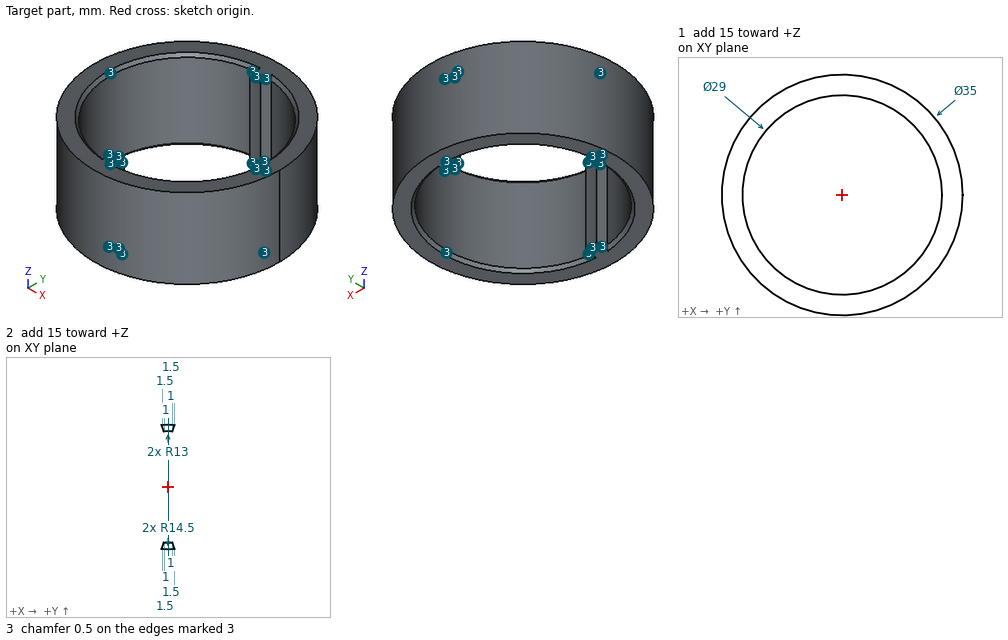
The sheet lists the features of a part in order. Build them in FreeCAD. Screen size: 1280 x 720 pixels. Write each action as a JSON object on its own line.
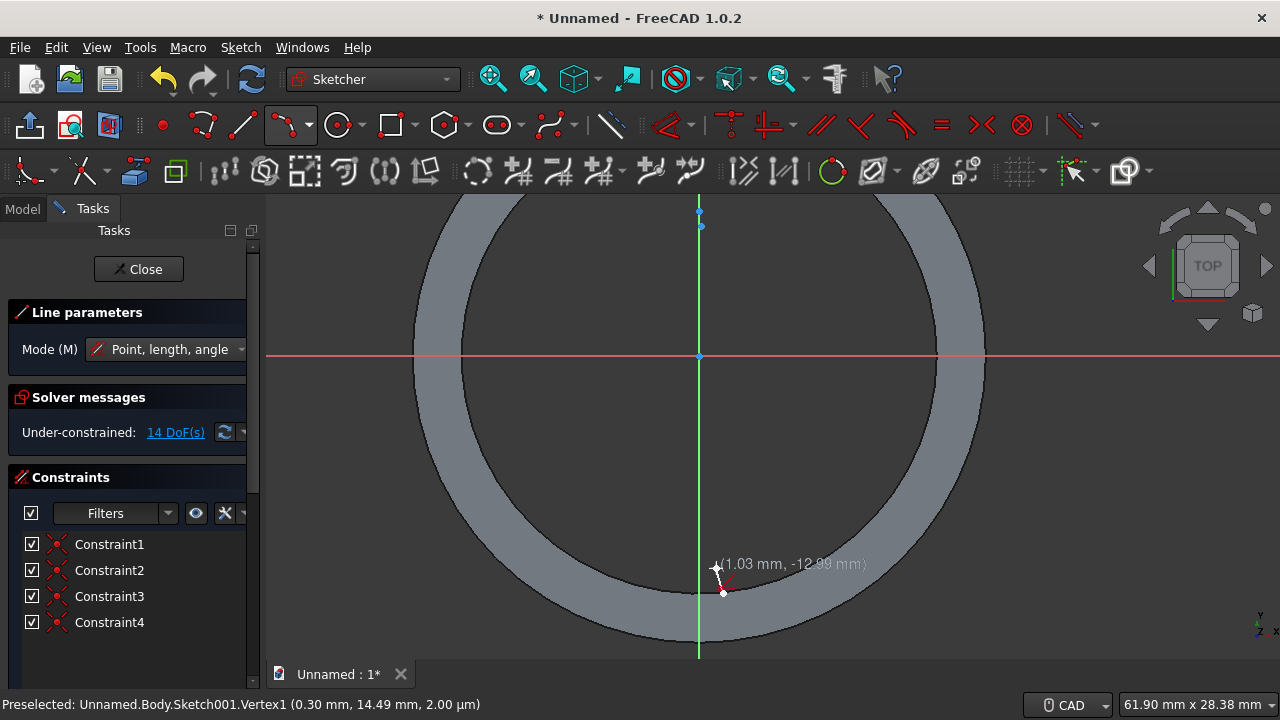
{"action": "left_click", "coordinate": [683, 568]}
{"action": "left_click", "coordinate": [675, 592]}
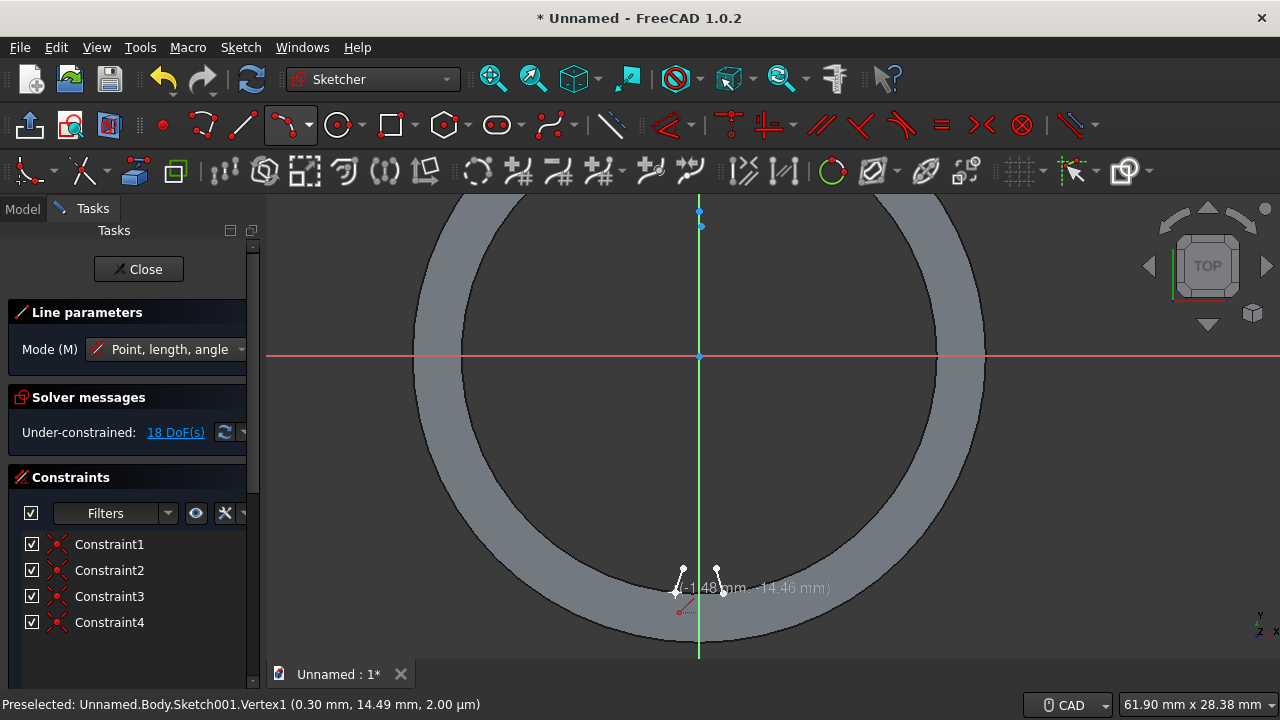
{"action": "left_click", "coordinate": [284, 126]}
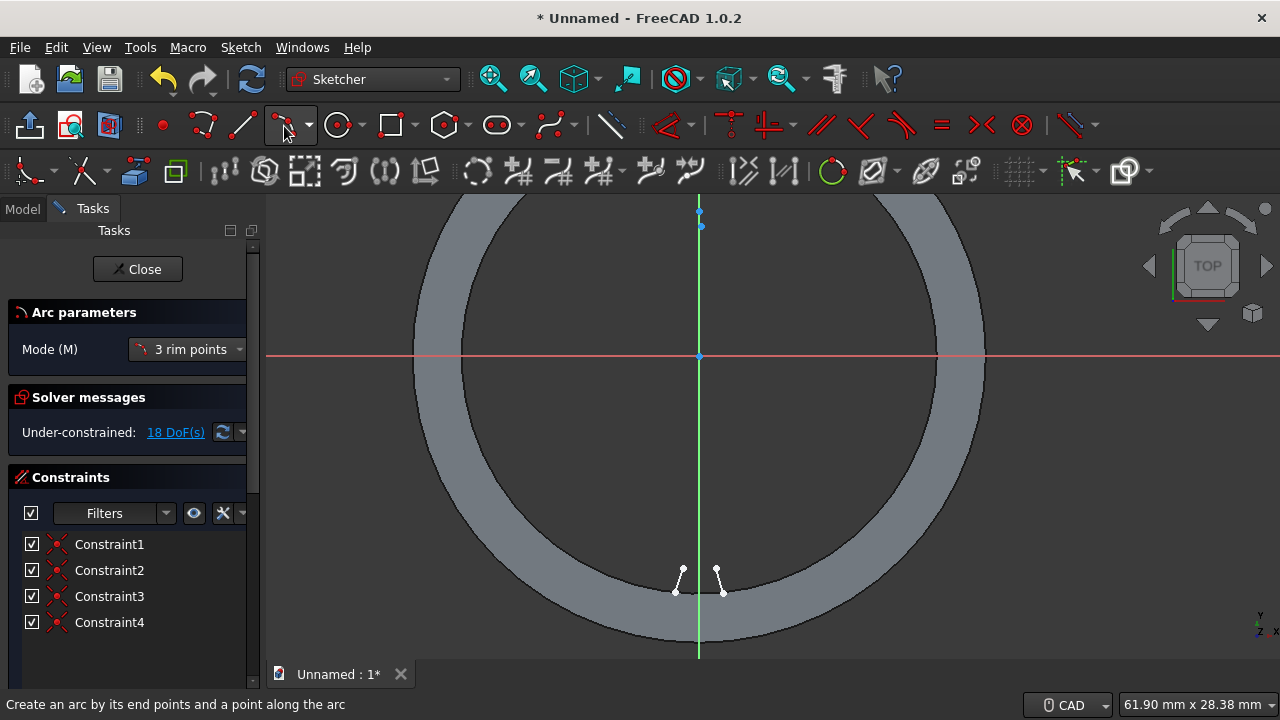
{"action": "scroll", "coordinate": [716, 568], "scroll_direction": "up", "scroll_amount": 2}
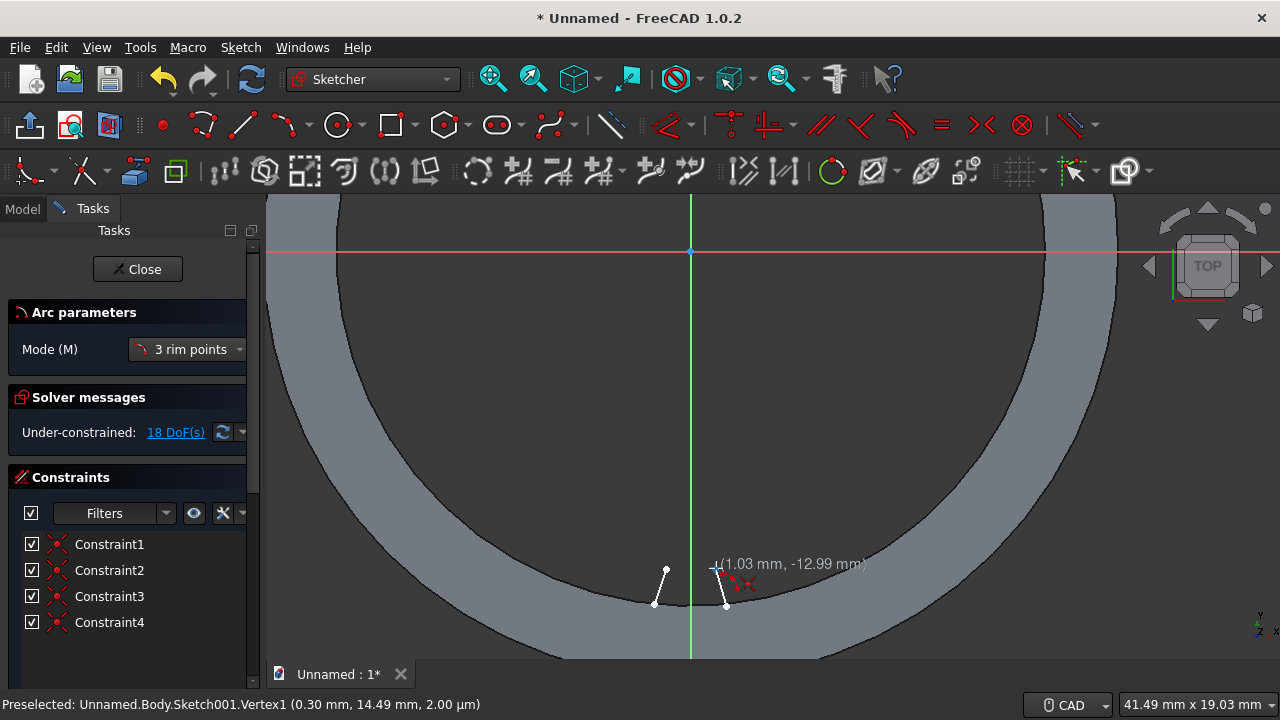
{"action": "left_click", "coordinate": [716, 569]}
{"action": "left_click", "coordinate": [667, 569]}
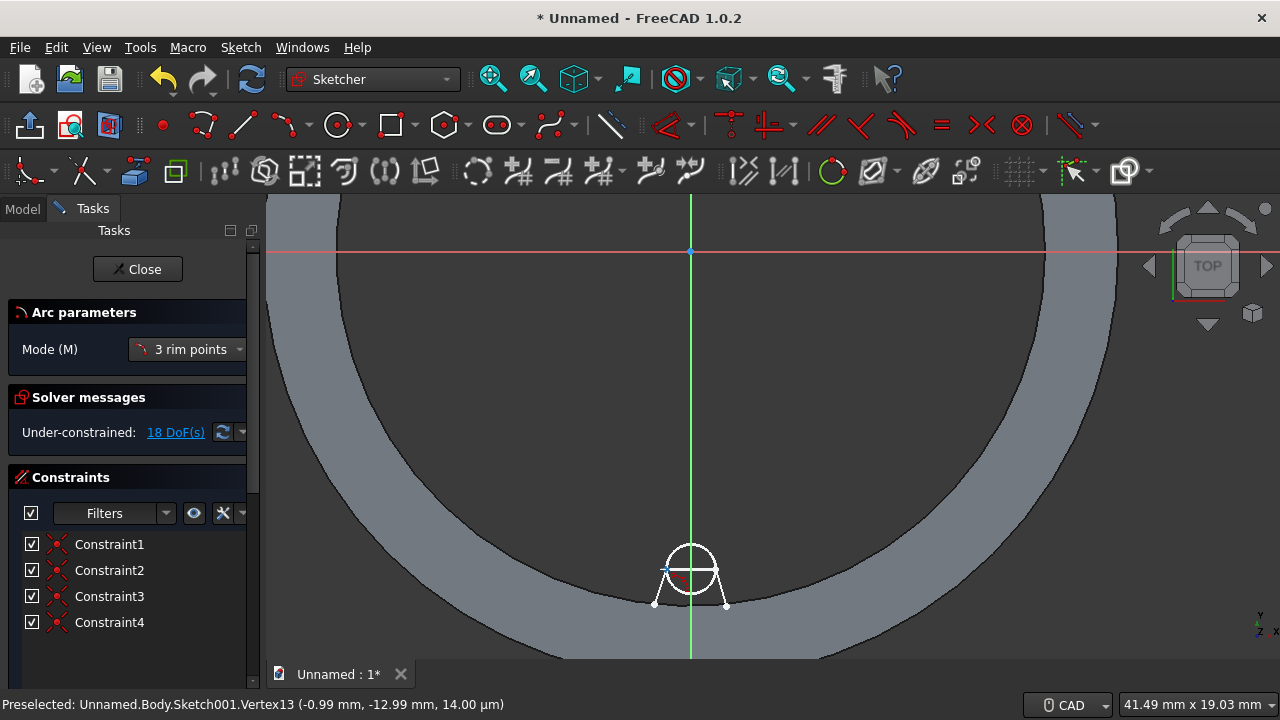
{"action": "scroll", "coordinate": [686, 569], "scroll_direction": "up", "scroll_amount": 15}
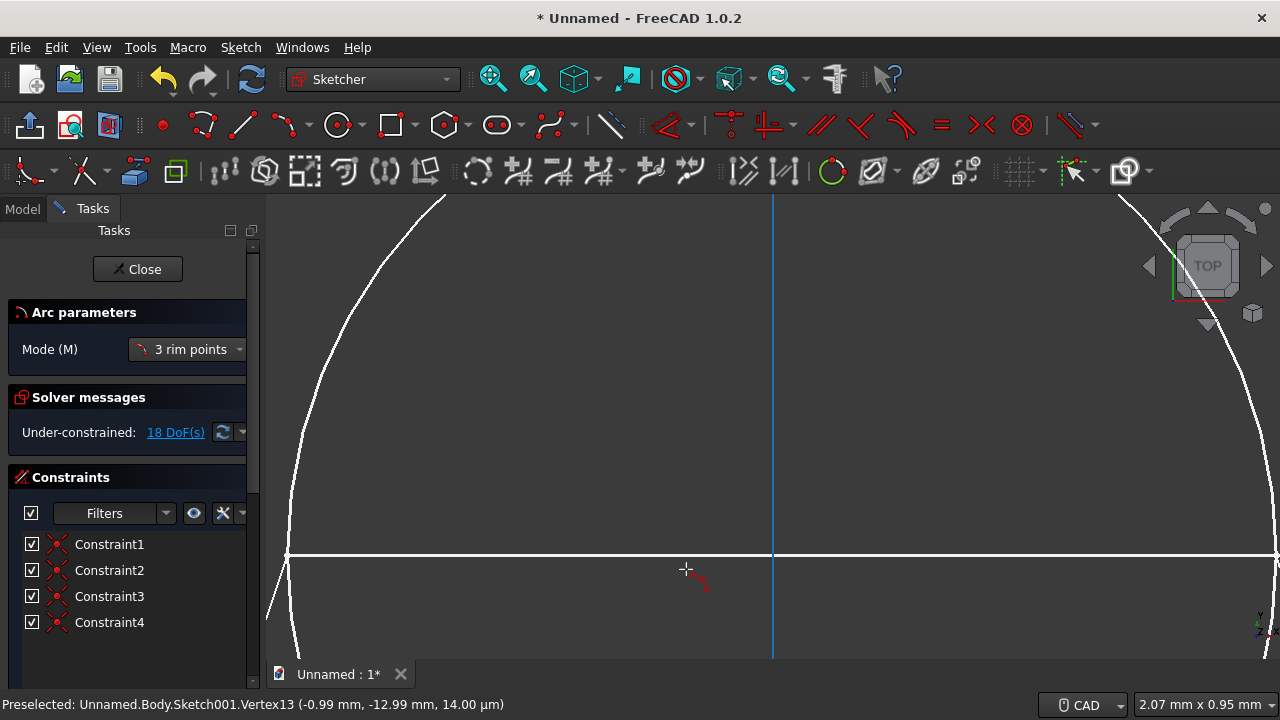
{"action": "left_click", "coordinate": [674, 557]}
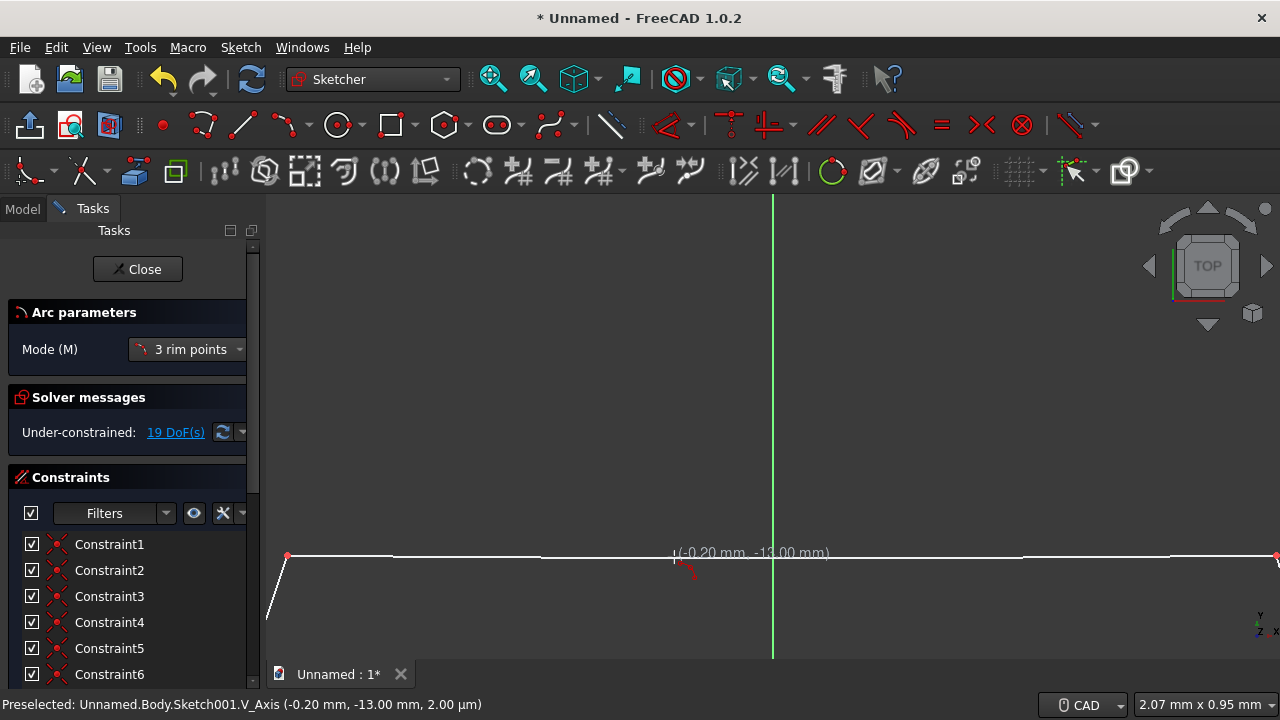
{"action": "scroll", "coordinate": [704, 426], "scroll_direction": "down", "scroll_amount": 15}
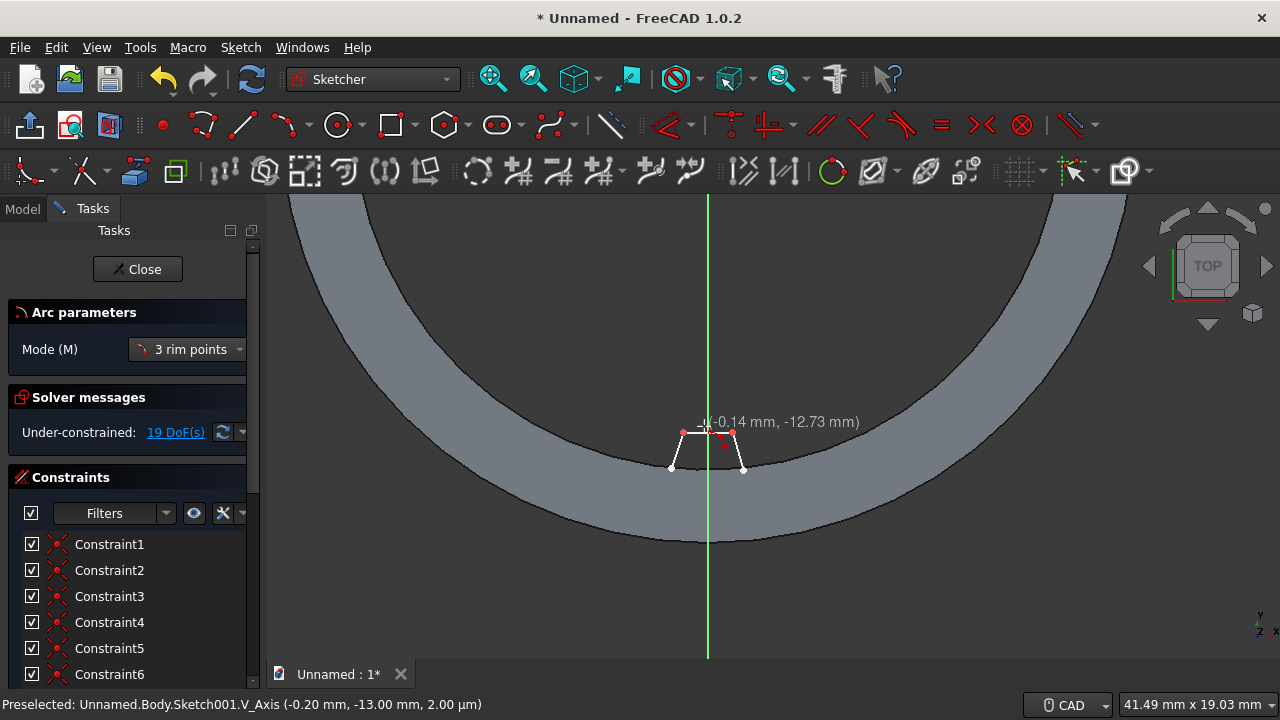
{"action": "scroll", "coordinate": [703, 608], "scroll_direction": "down", "scroll_amount": 5}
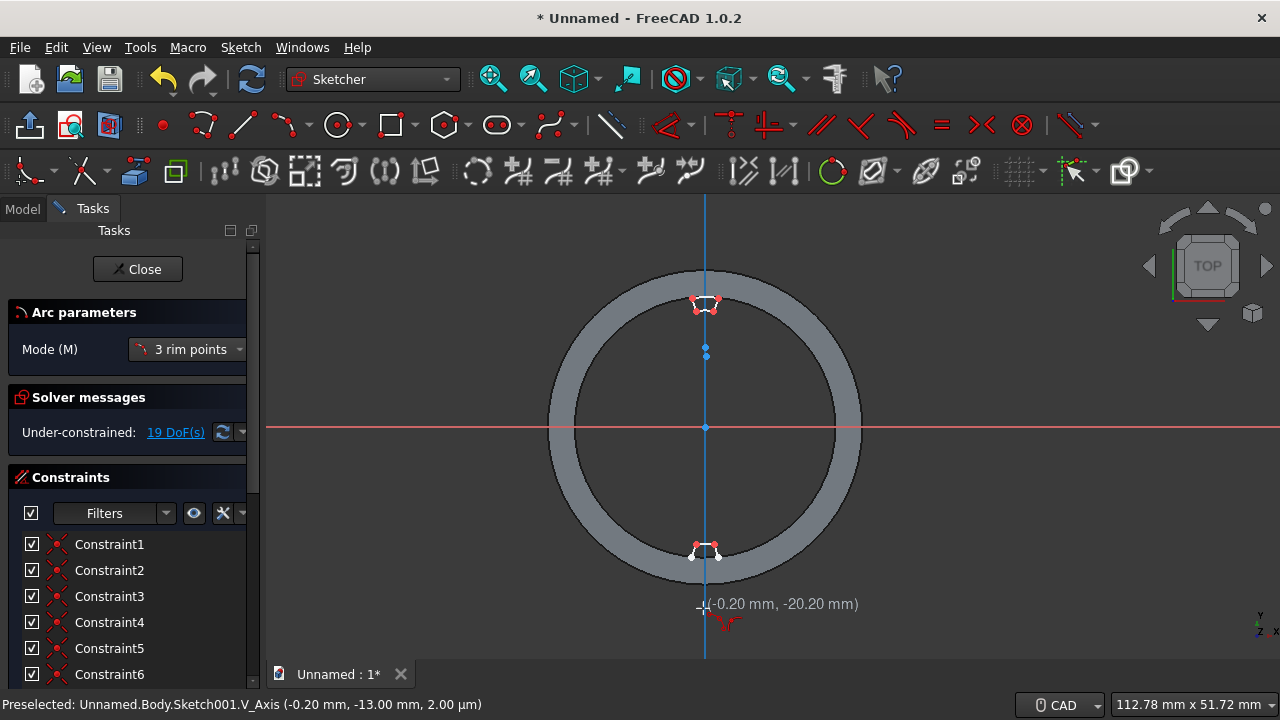
{"action": "scroll", "coordinate": [692, 557], "scroll_direction": "up", "scroll_amount": 5}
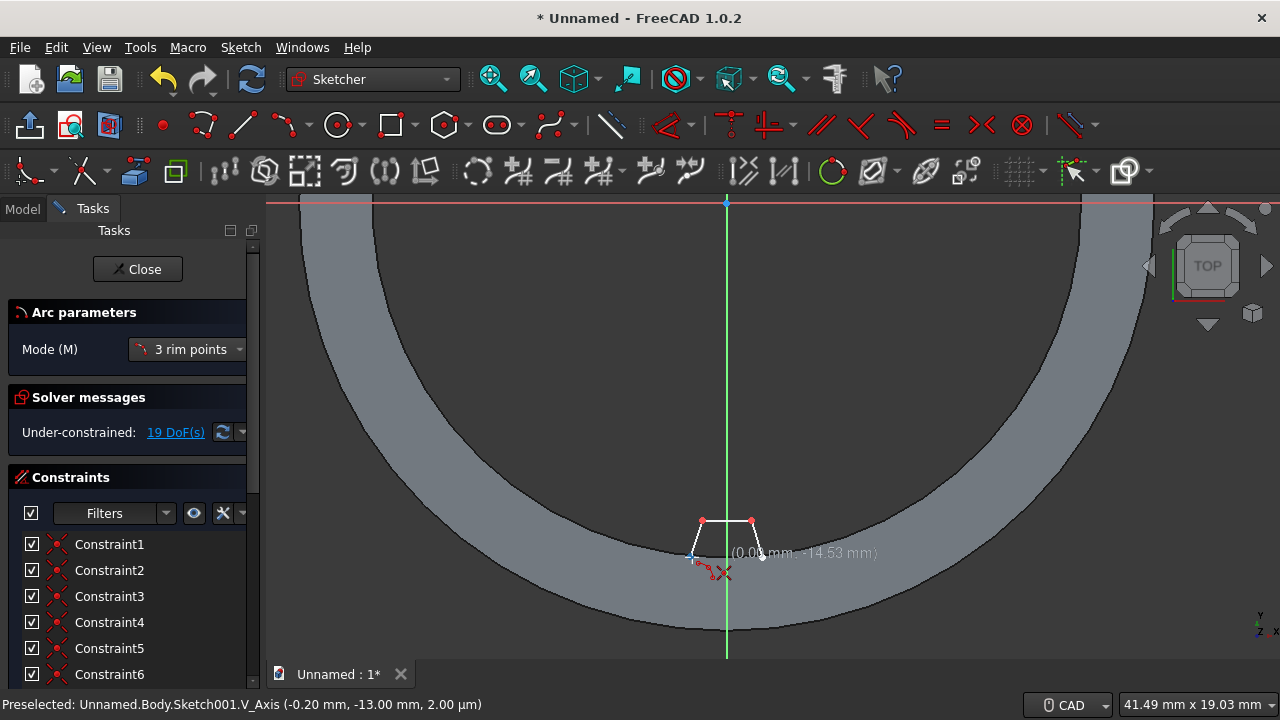
{"action": "left_click", "coordinate": [691, 557]}
{"action": "left_click", "coordinate": [763, 558]}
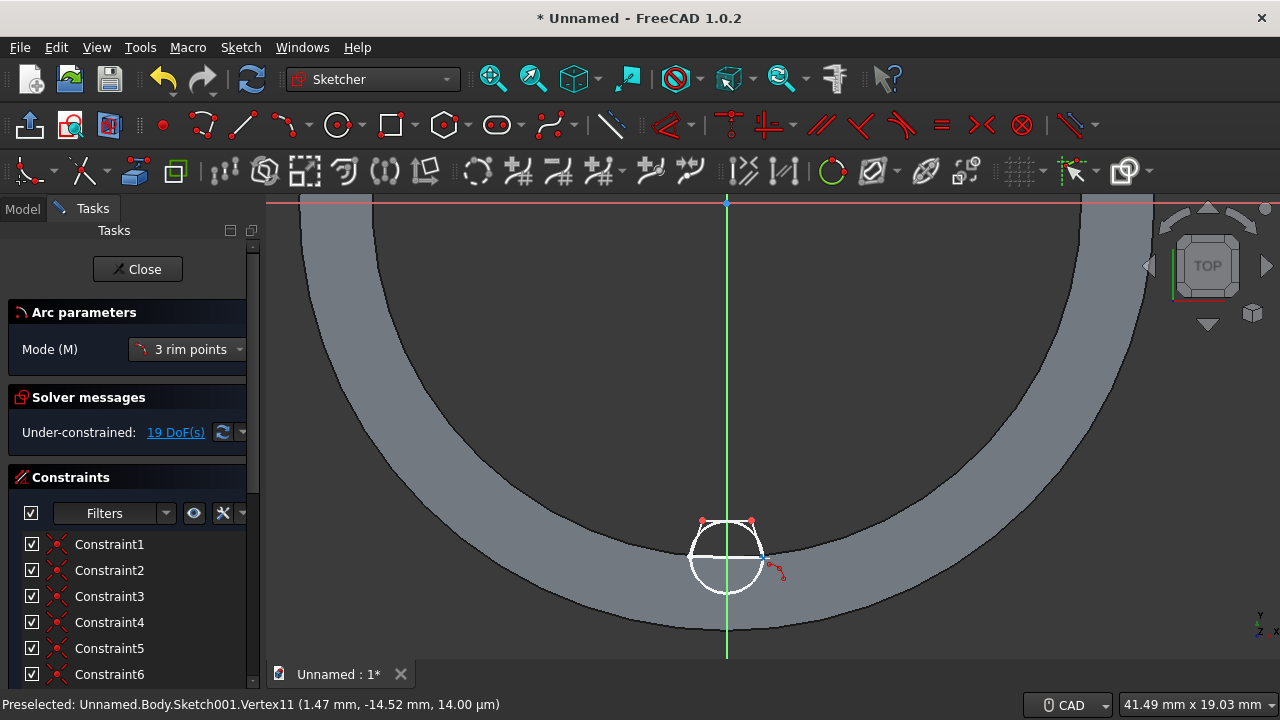
{"action": "scroll", "coordinate": [719, 557], "scroll_direction": "up", "scroll_amount": 11}